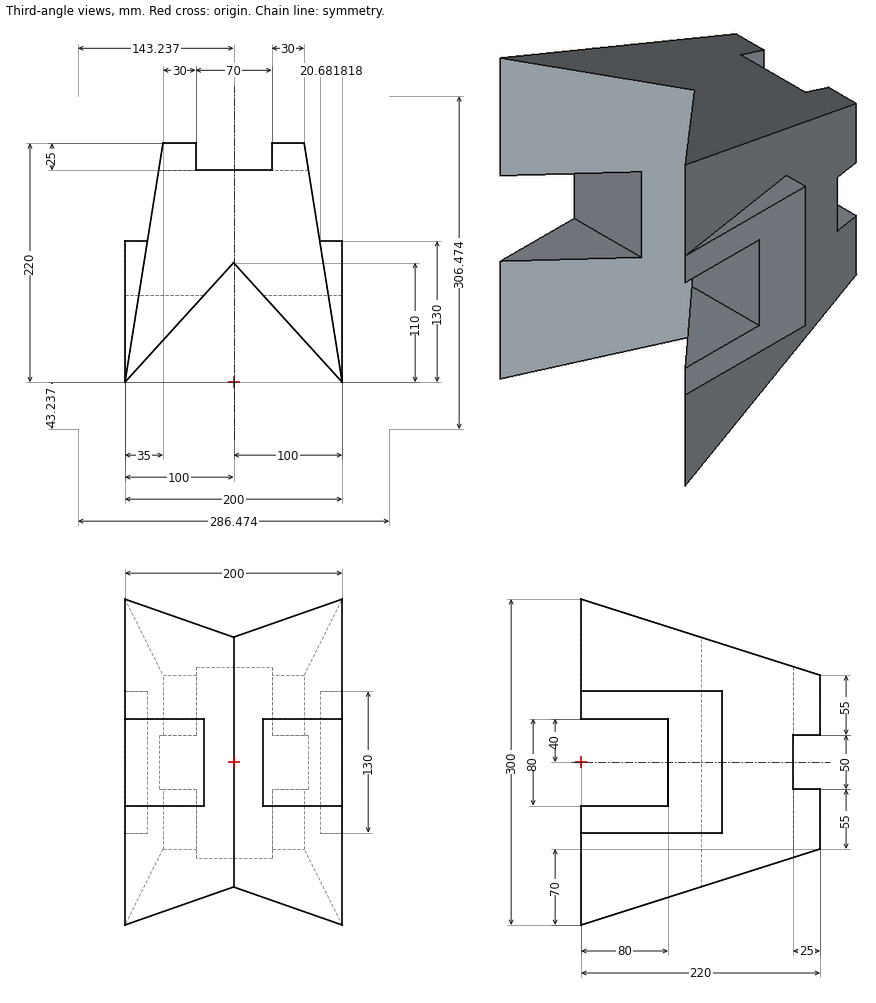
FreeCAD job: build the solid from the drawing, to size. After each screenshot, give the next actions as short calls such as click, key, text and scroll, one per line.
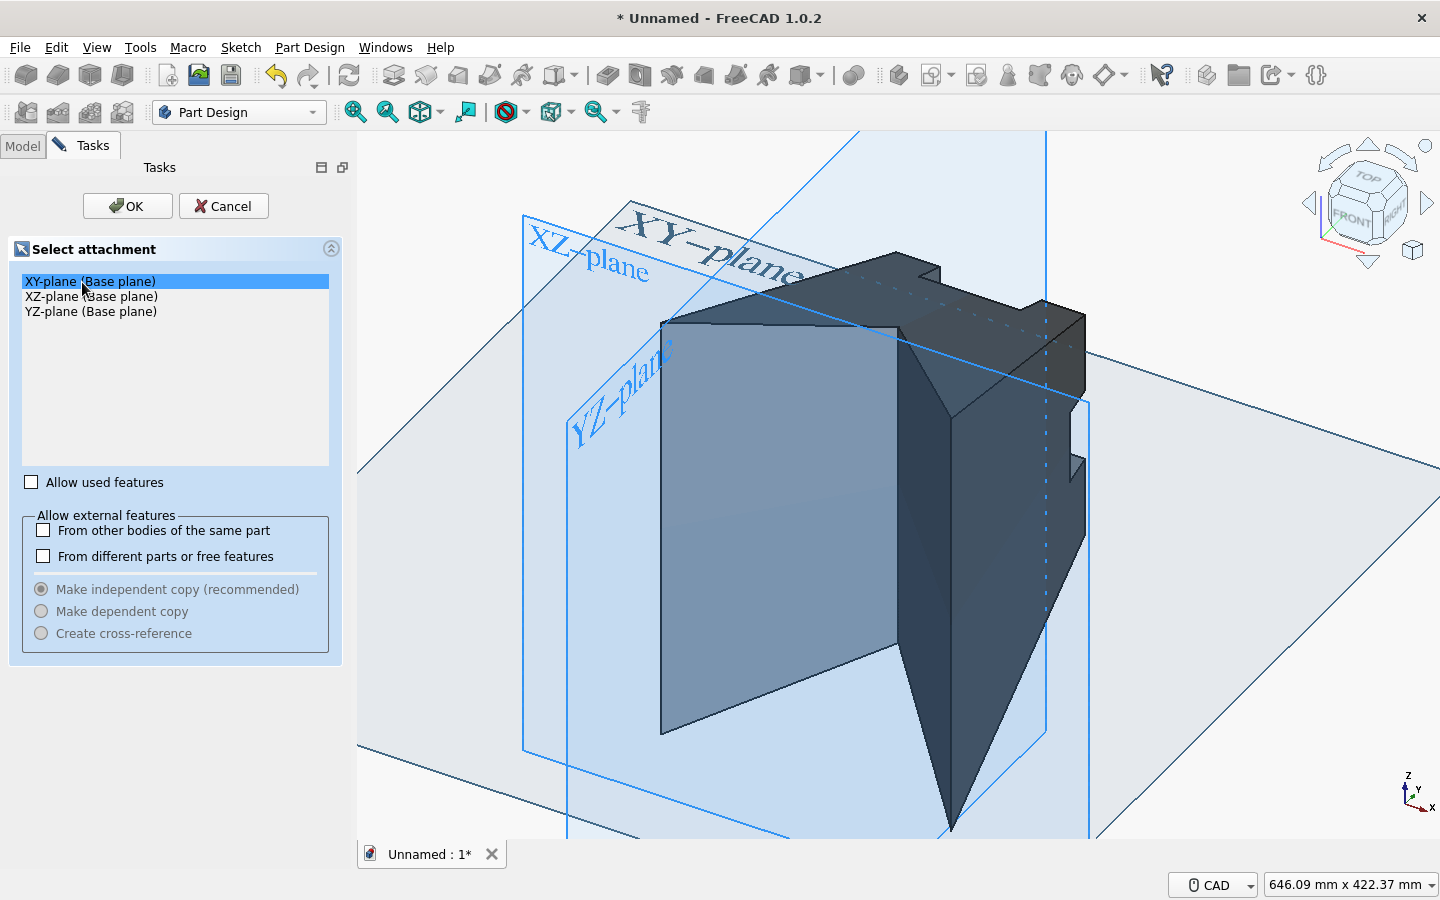
click(128, 206)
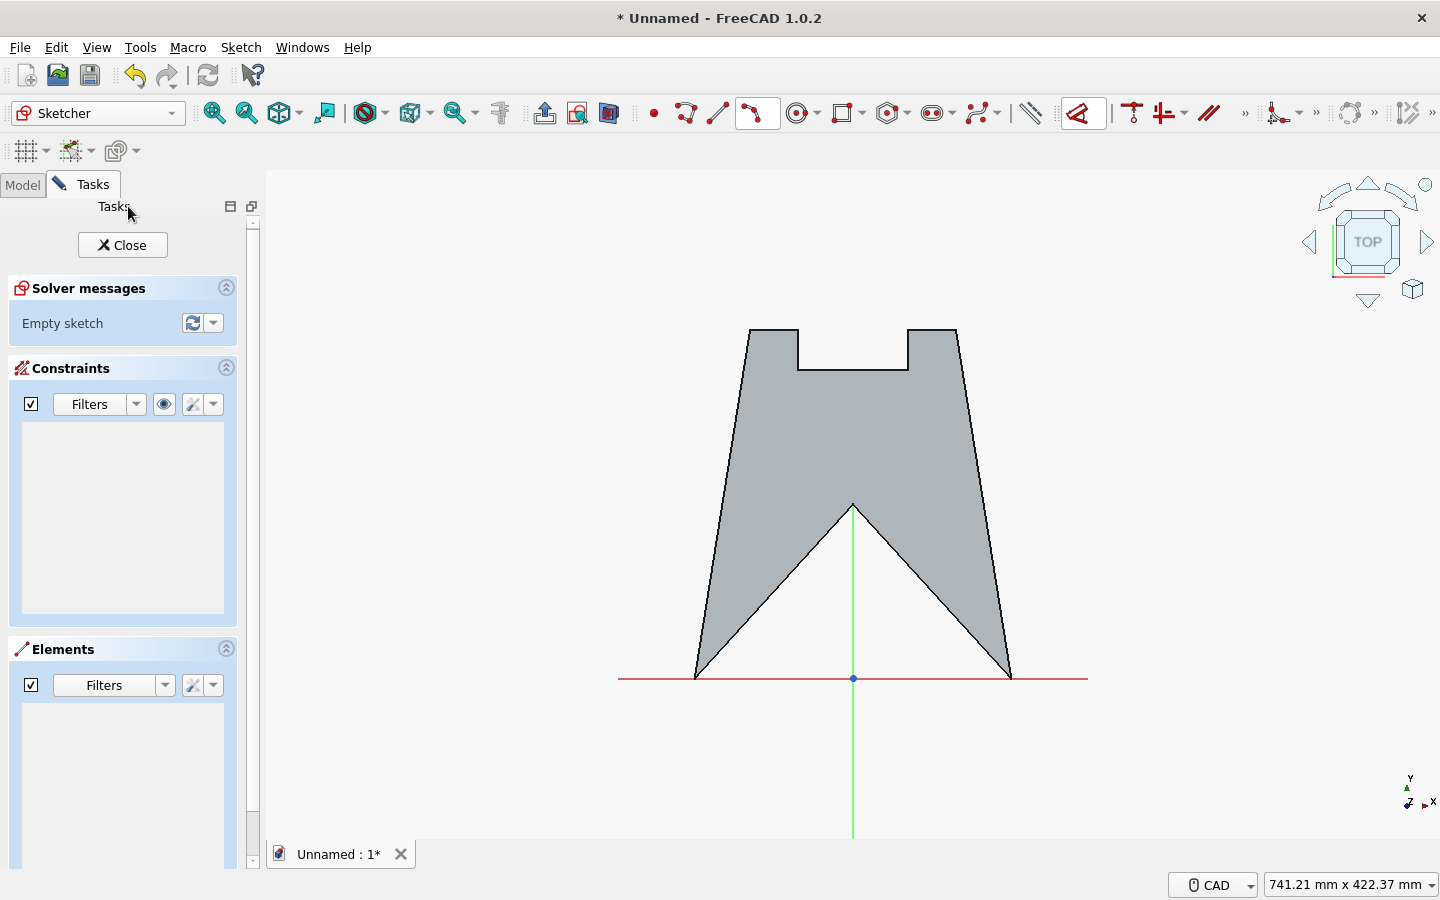
key(q)
key(s)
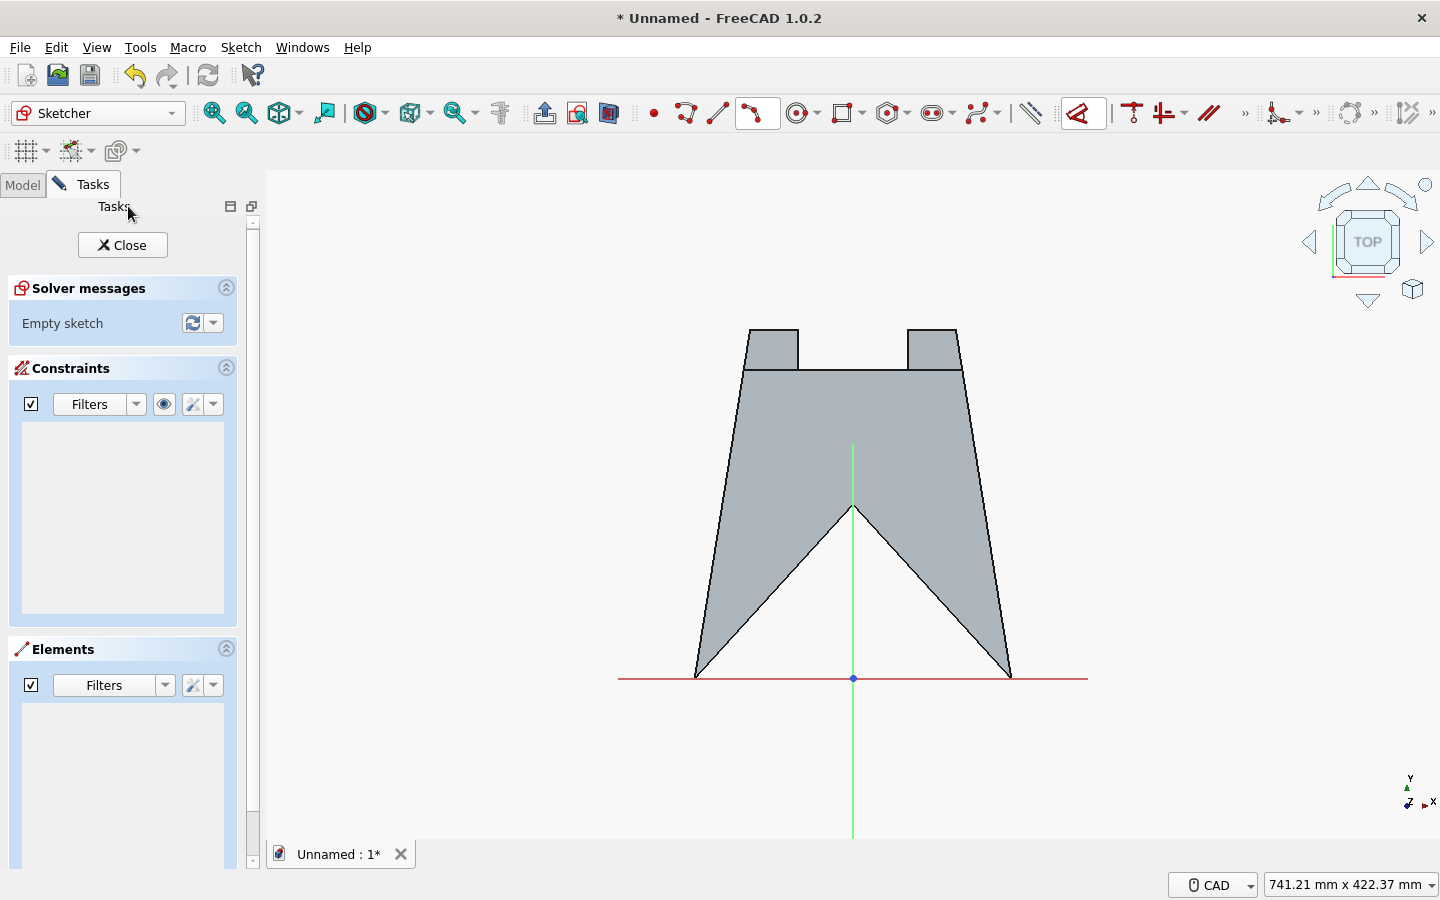
scroll(1053, 634, up, 4)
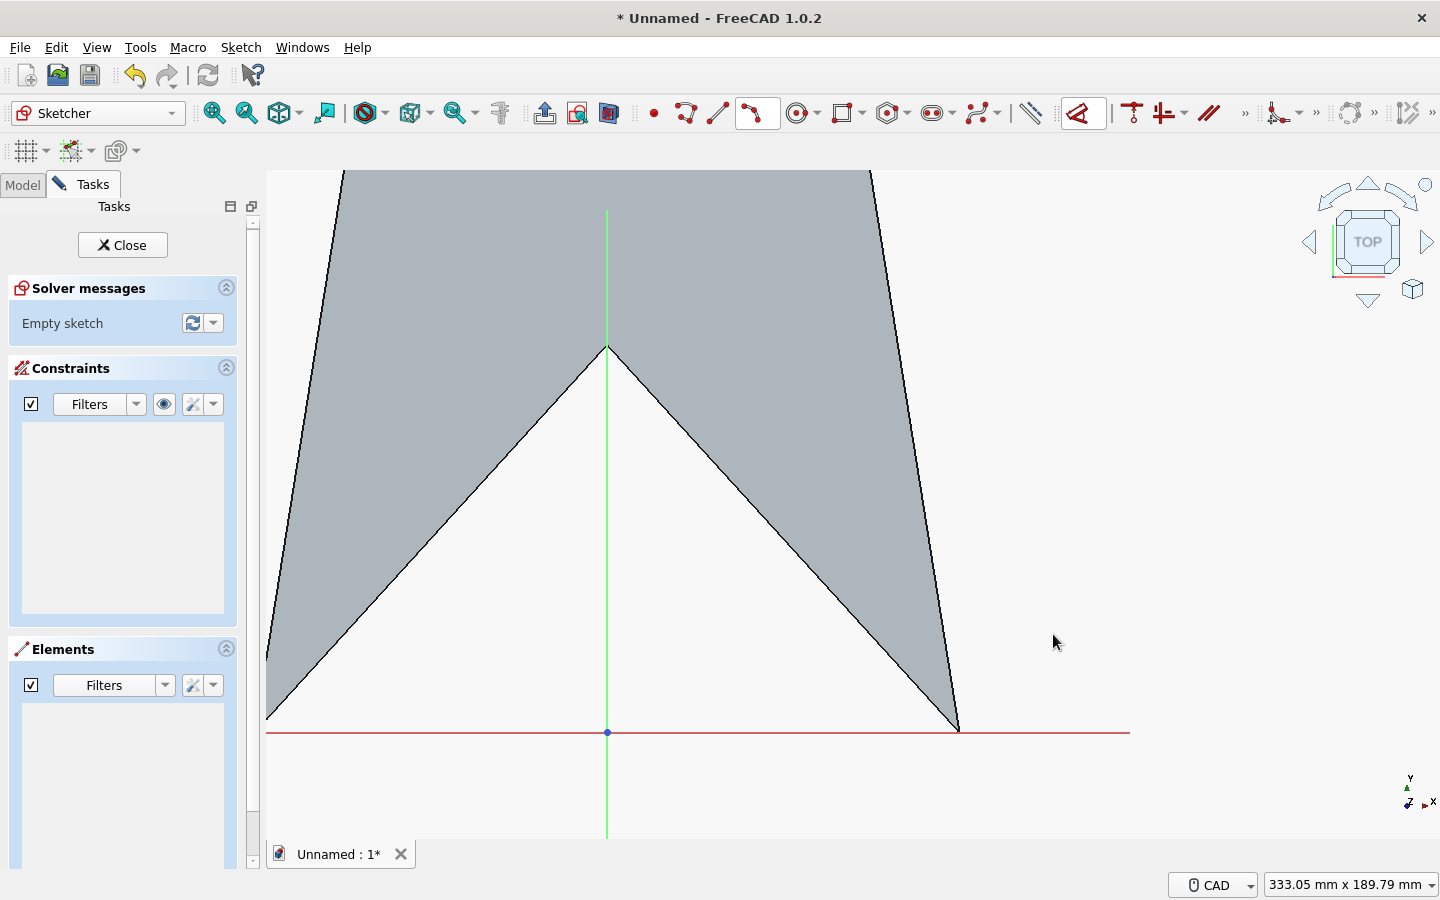
key(g)
key(m)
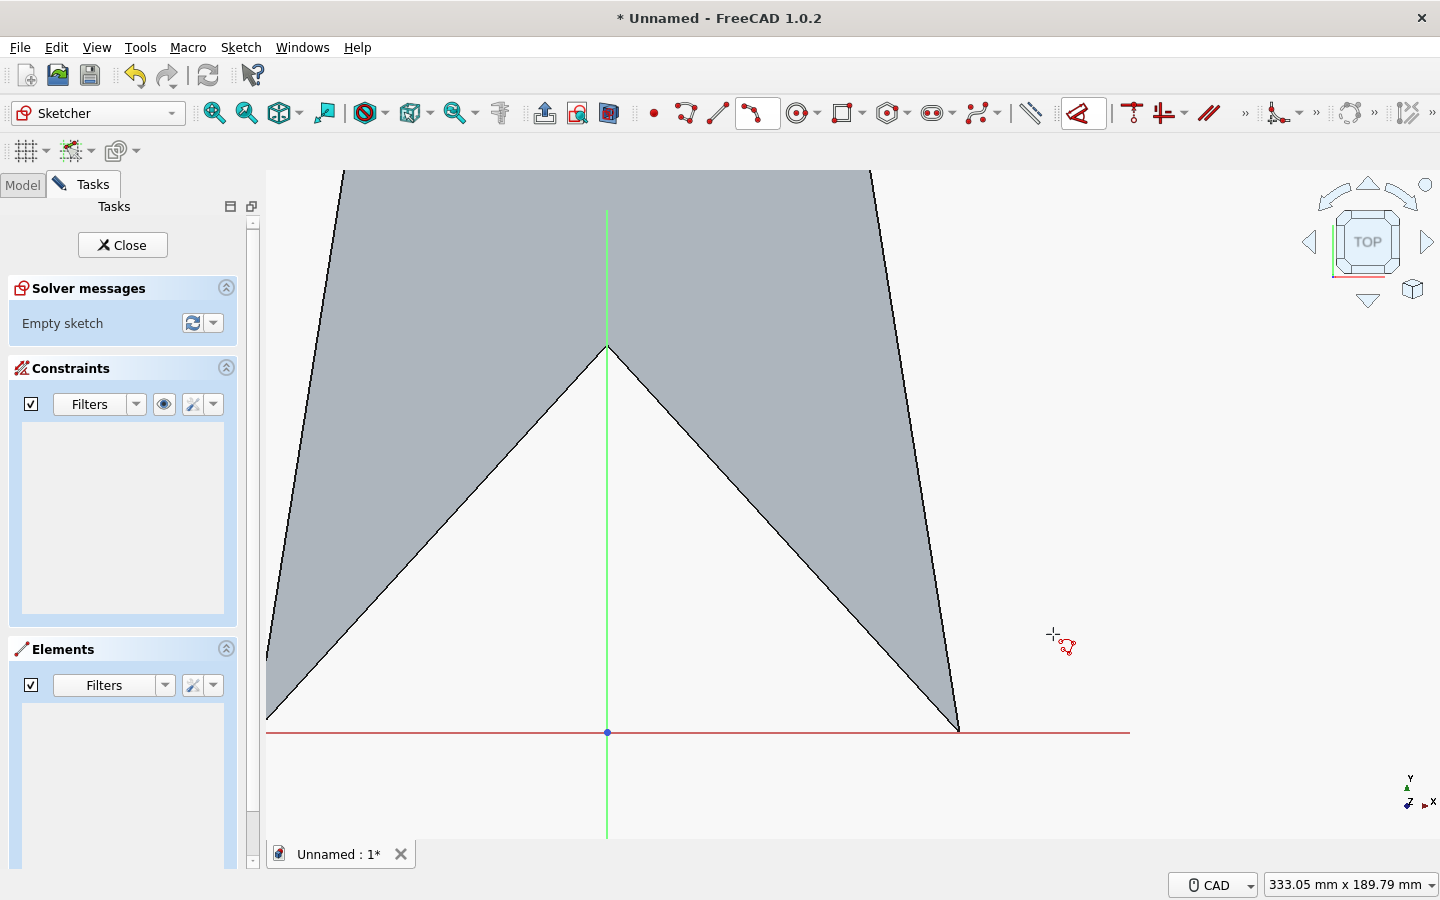
click(960, 733)
click(960, 274)
click(887, 274)
click(960, 733)
key(Escape)
key(Escape)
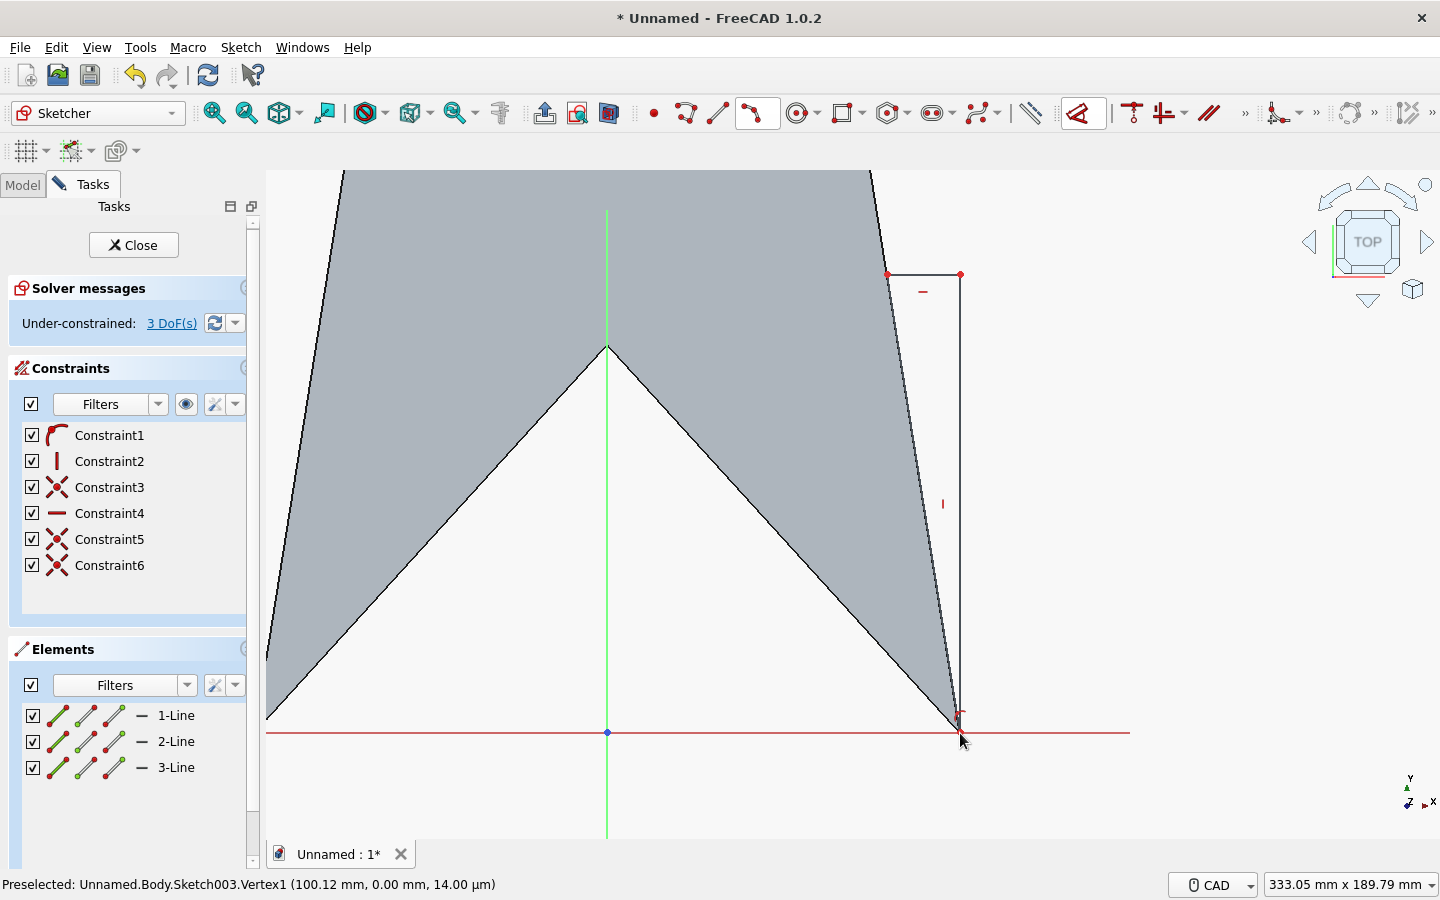
click(960, 595)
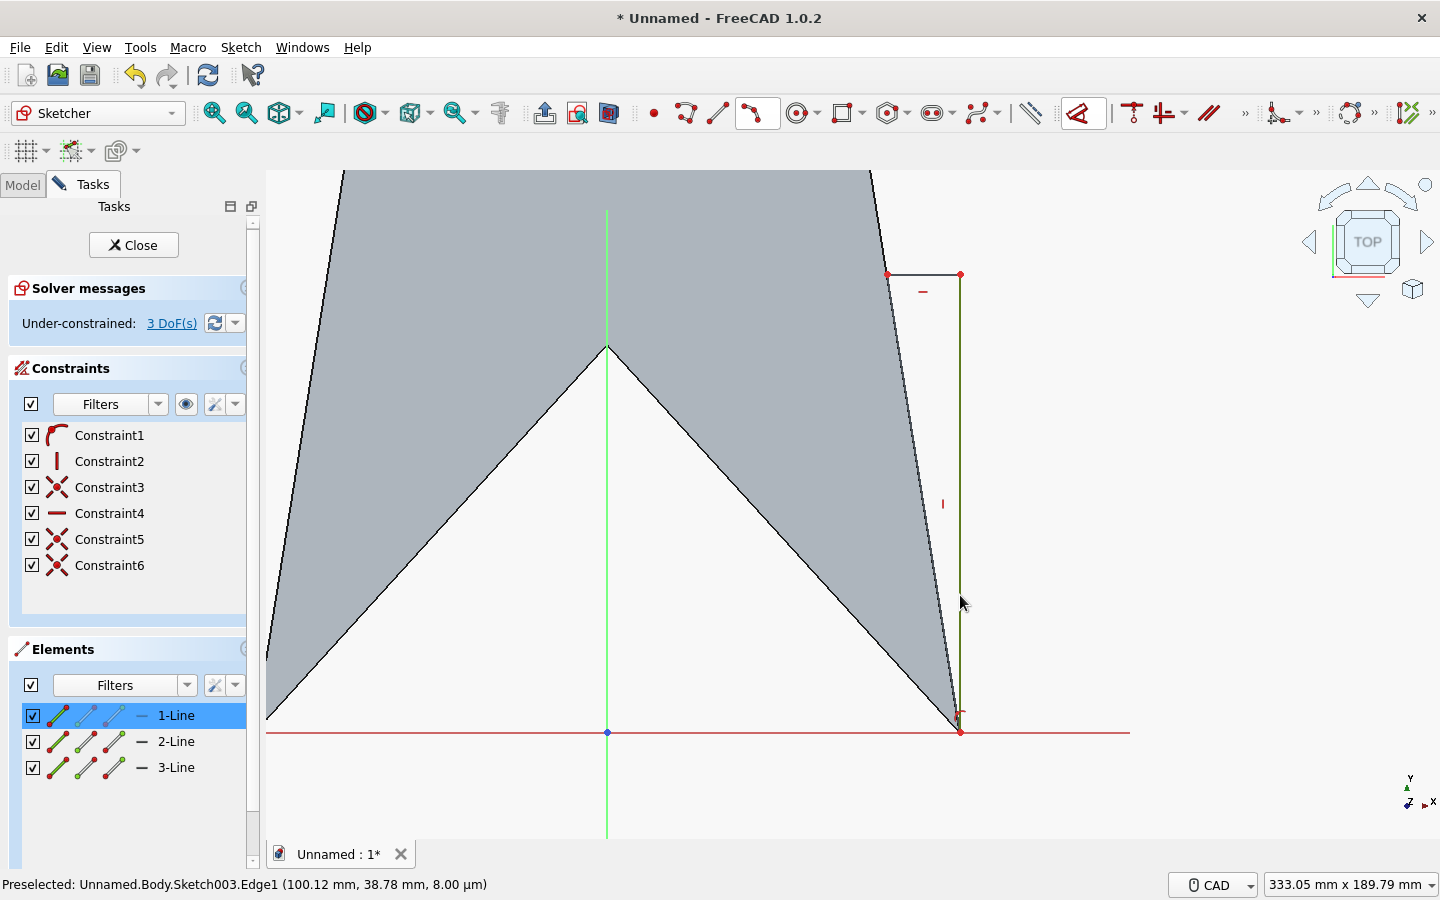
key(i)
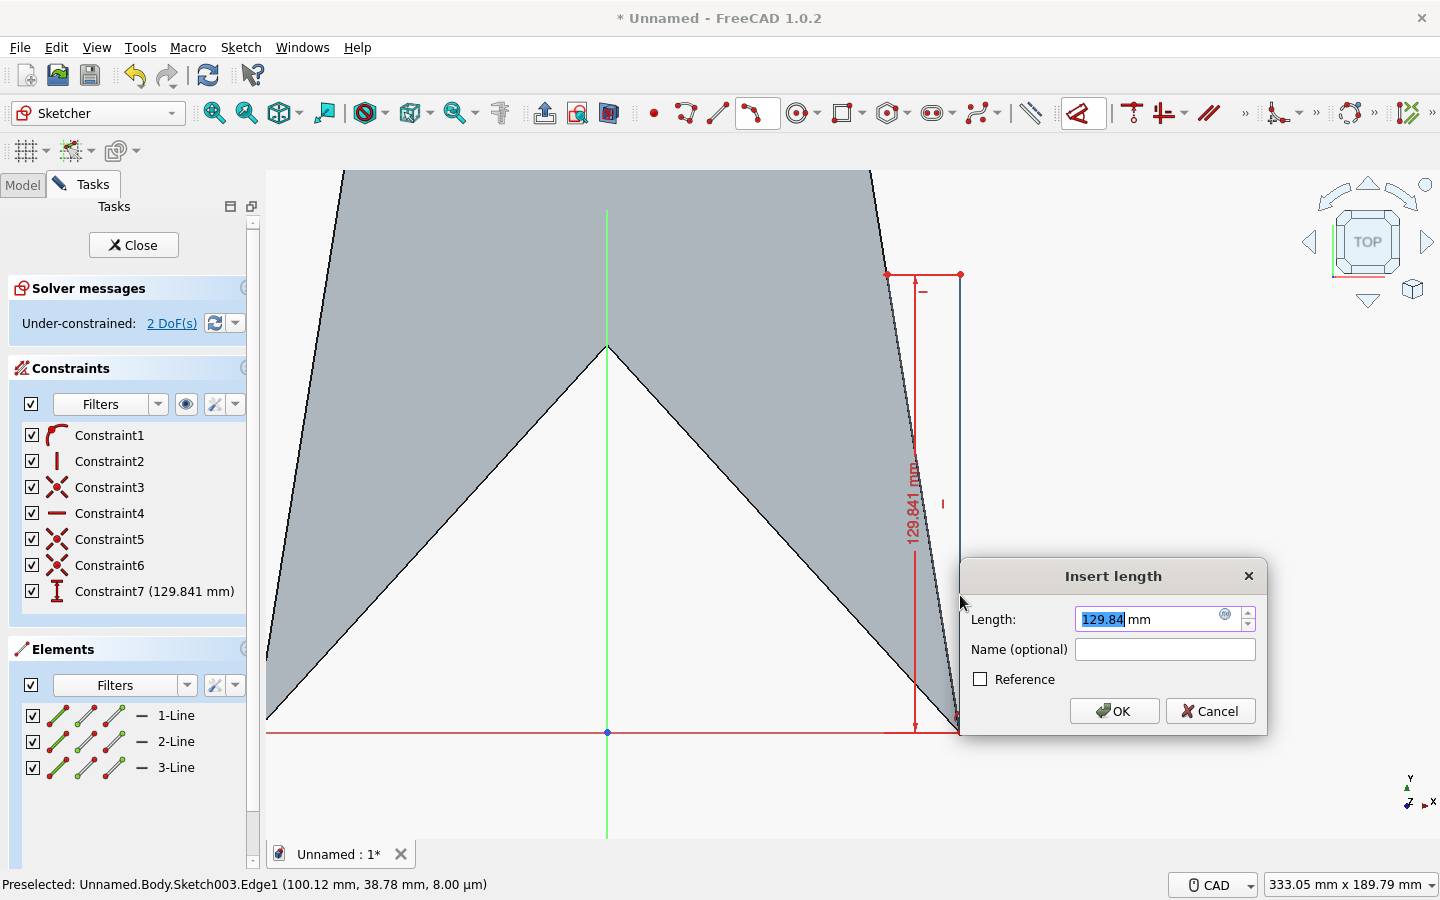
text(130)
key(Return)